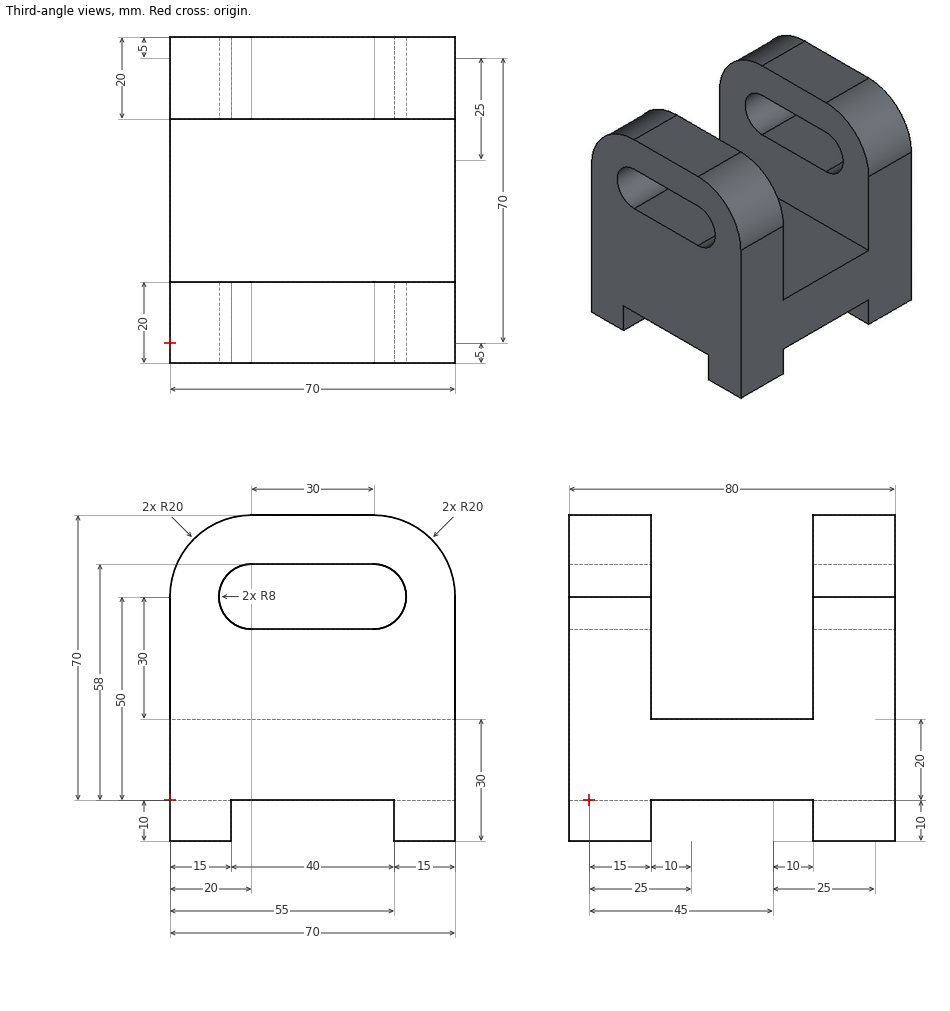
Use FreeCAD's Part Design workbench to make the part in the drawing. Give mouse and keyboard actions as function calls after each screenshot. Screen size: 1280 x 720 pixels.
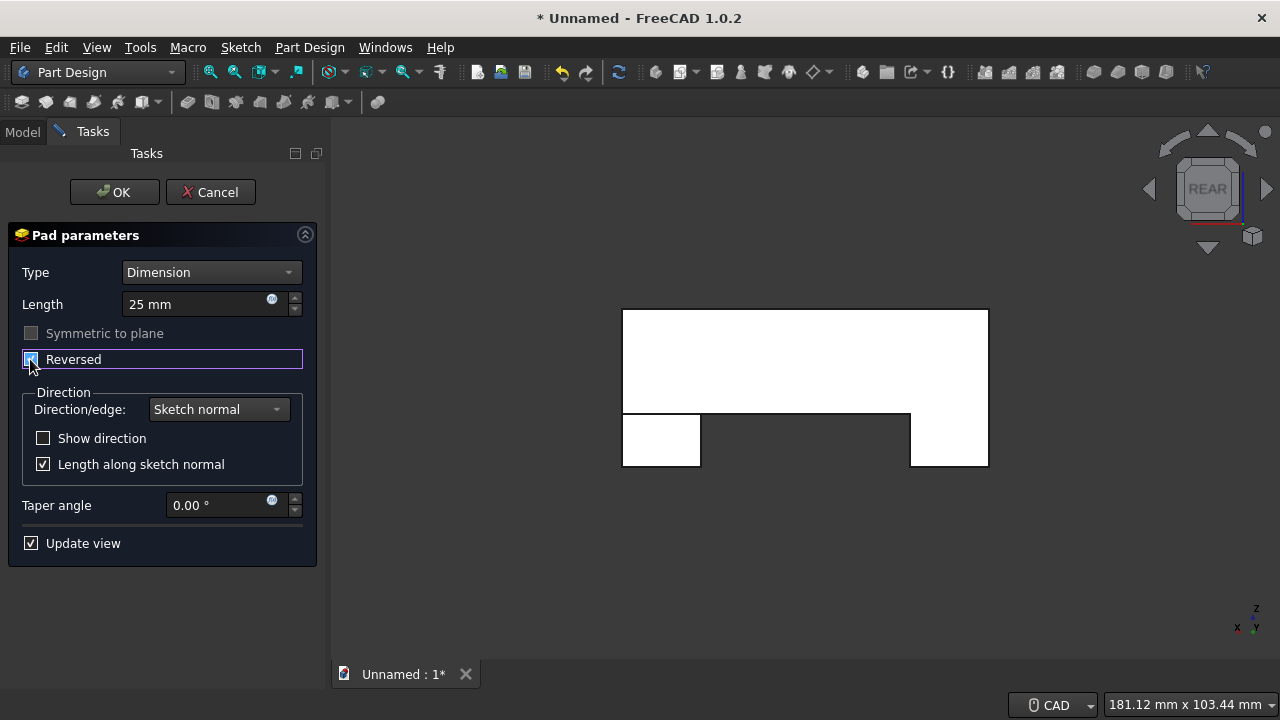
click(115, 192)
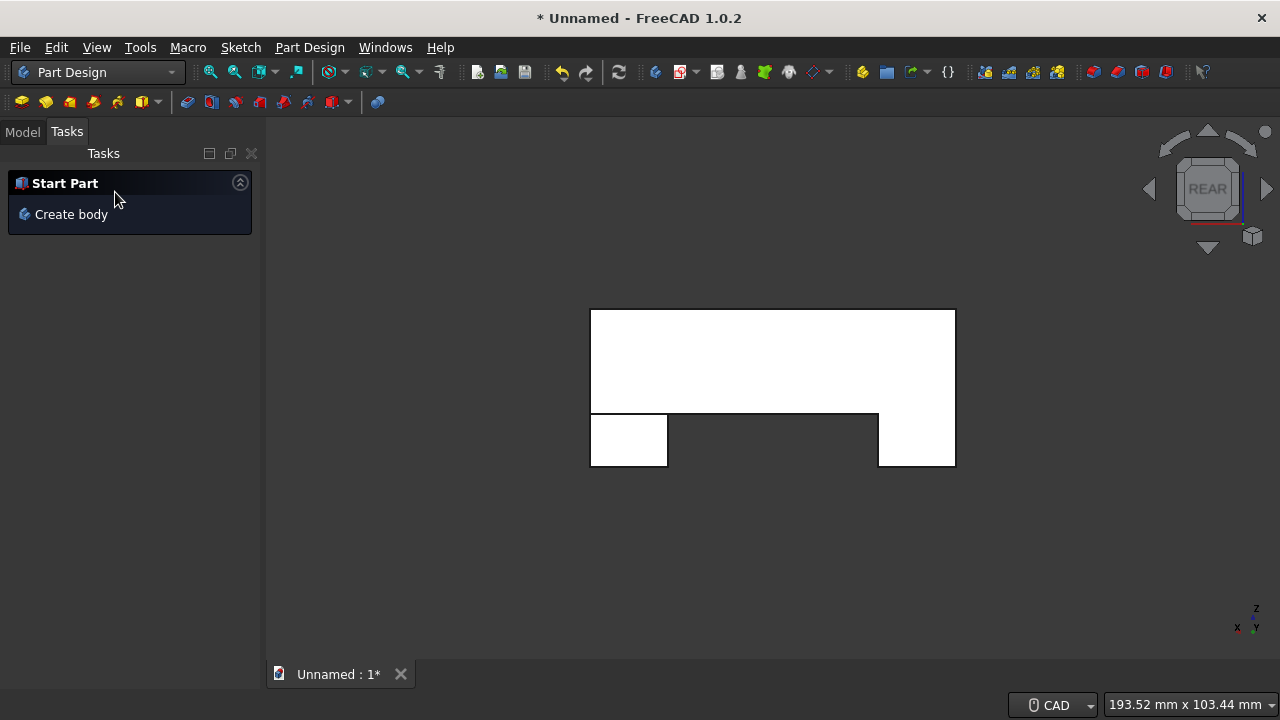
key(v)
key(f)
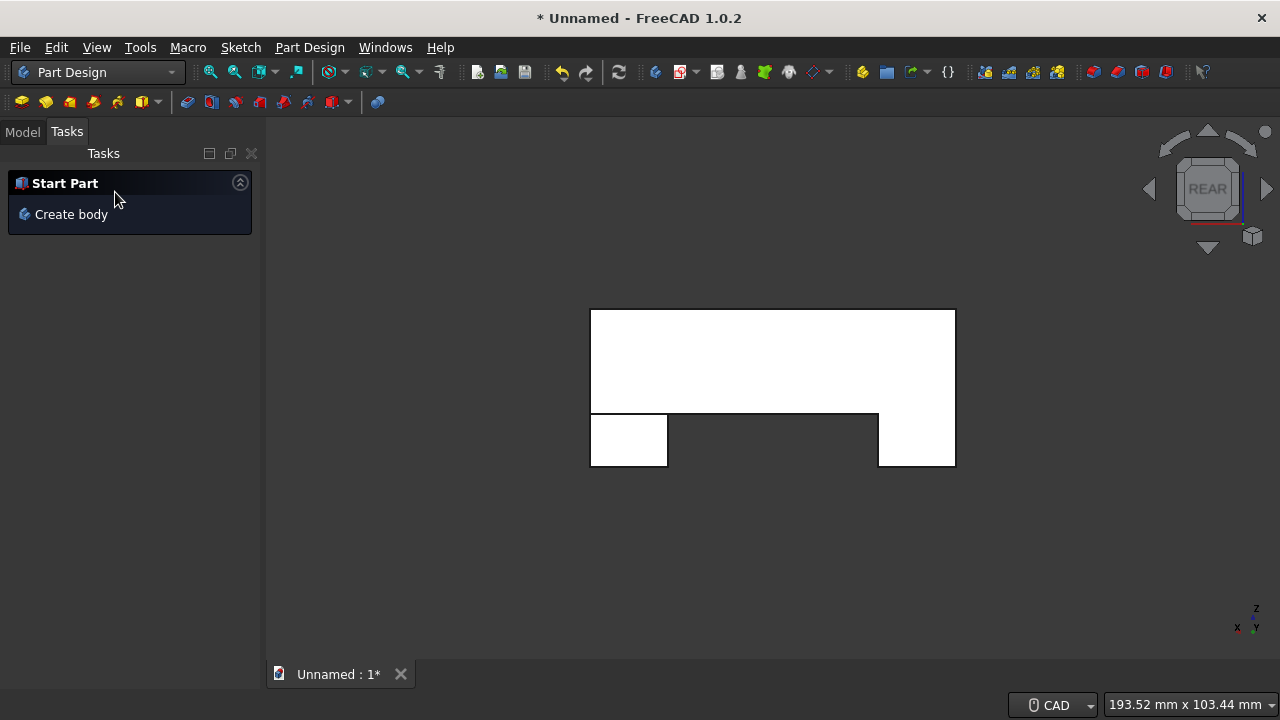
click(668, 365)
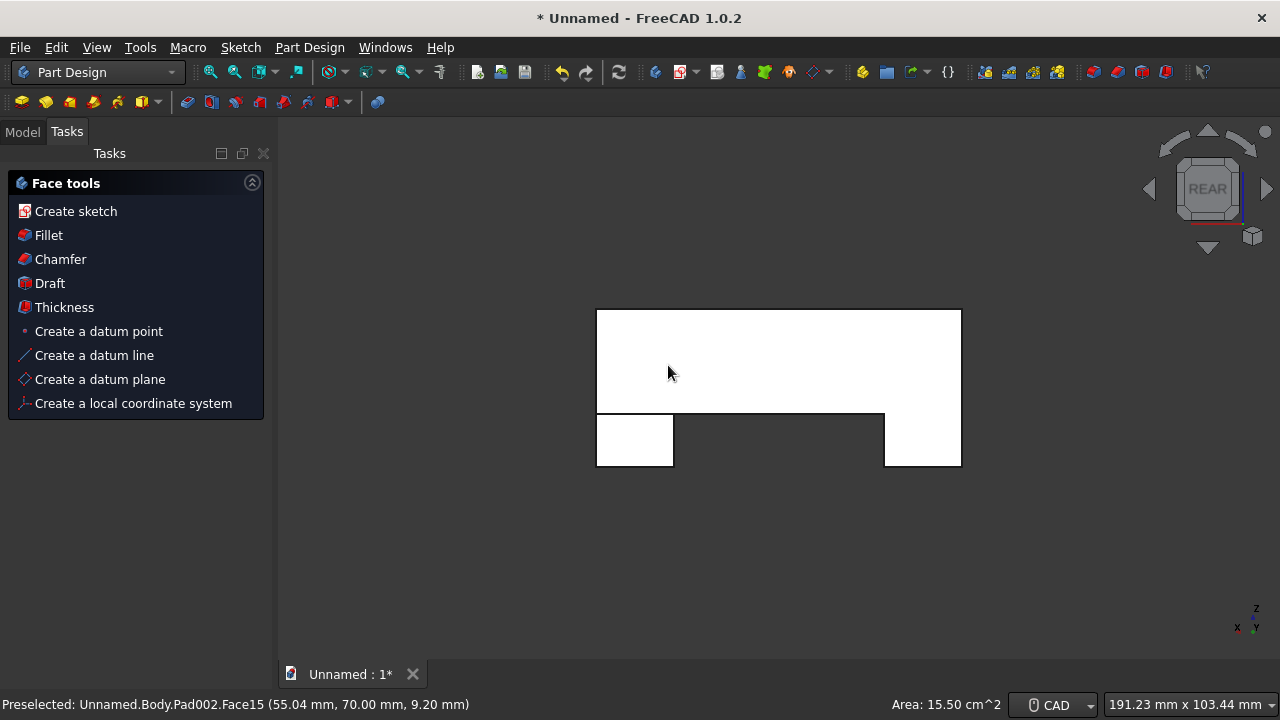
click(680, 72)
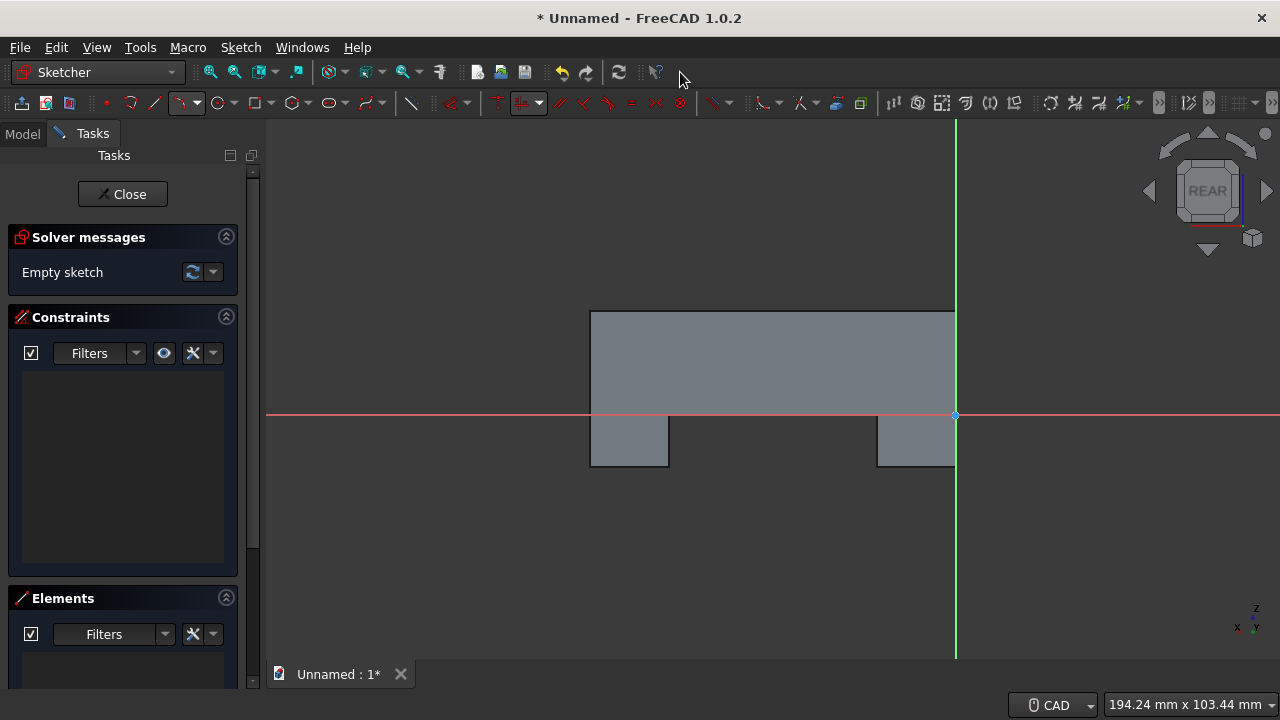
scroll(615, 452, up, 9)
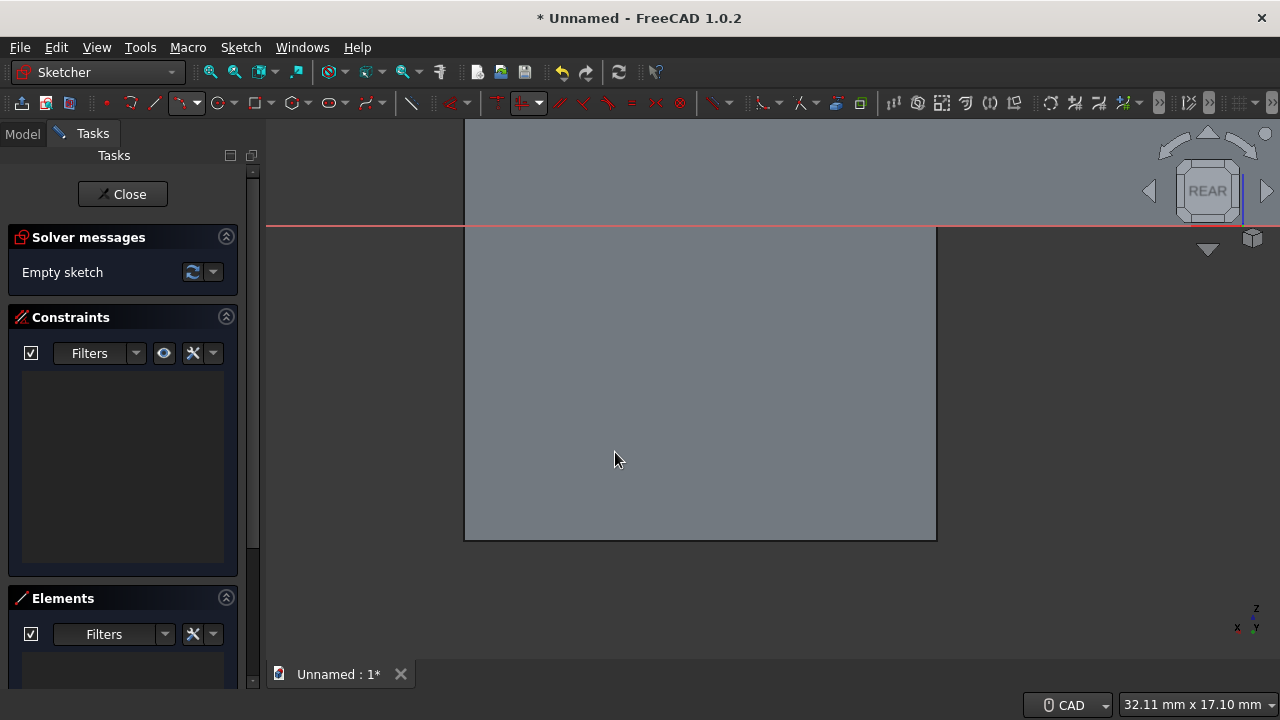
click(256, 104)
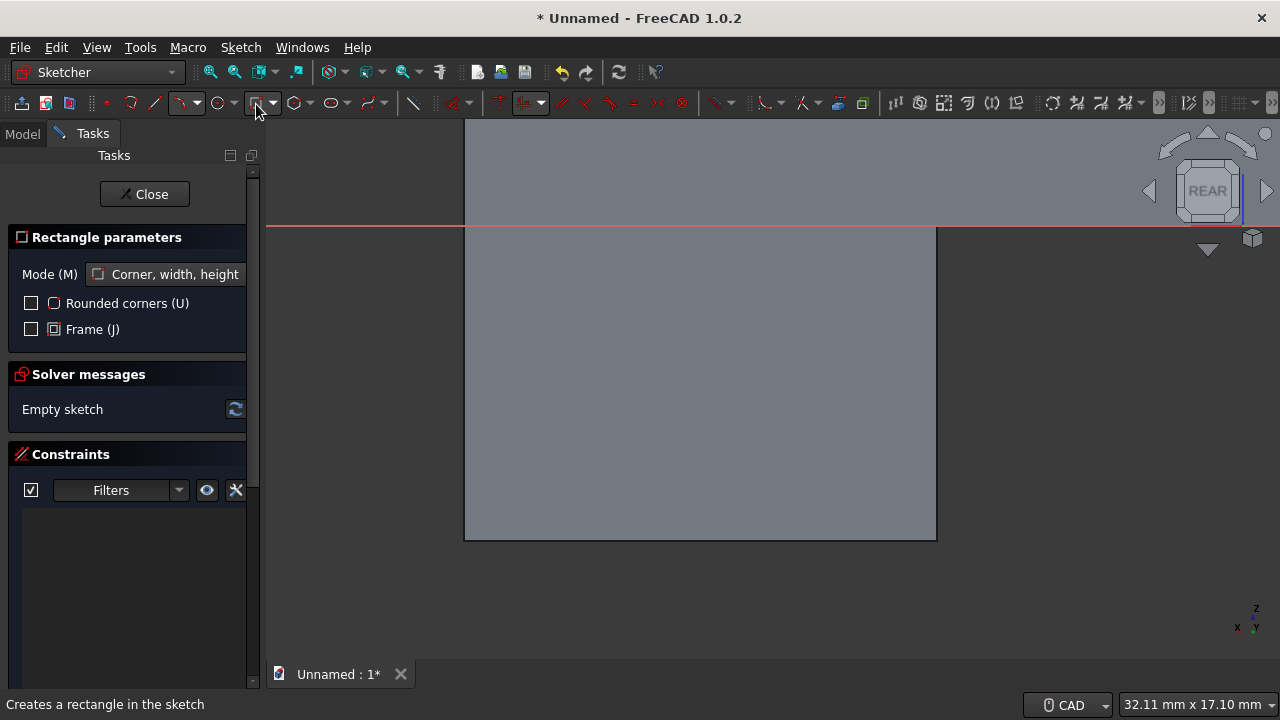
click(464, 226)
click(937, 541)
key(Escape)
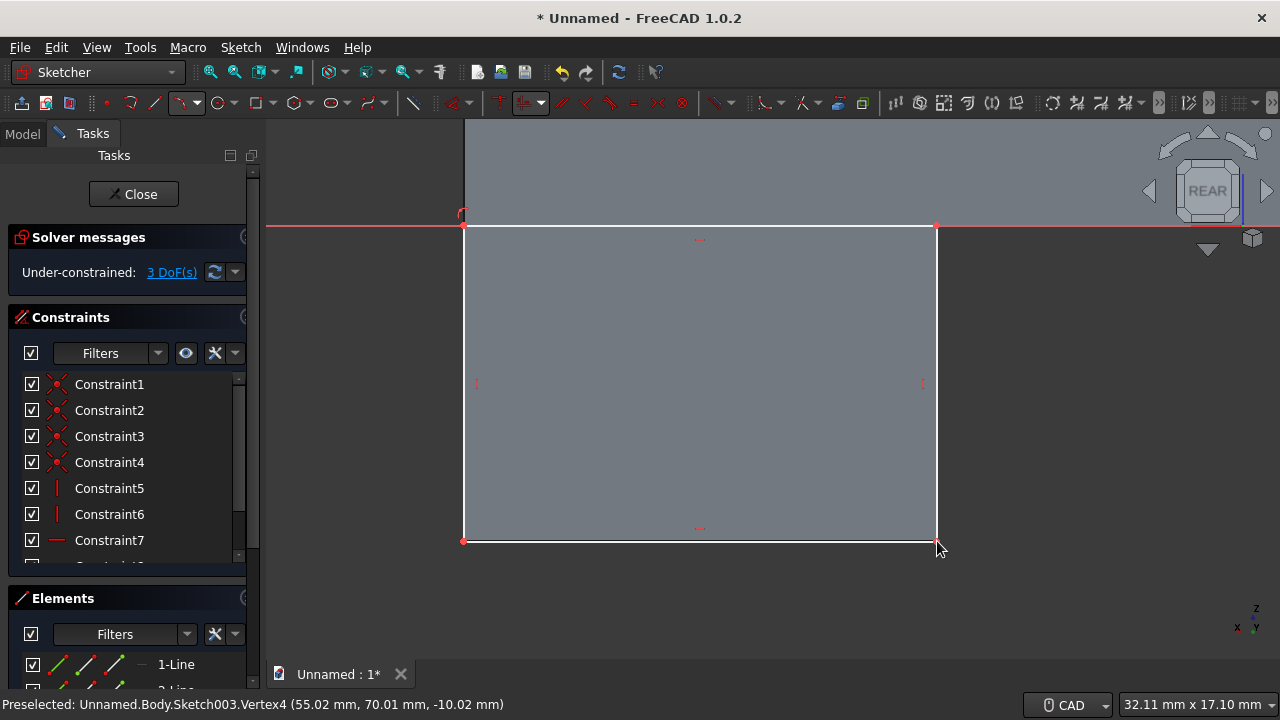
key(d)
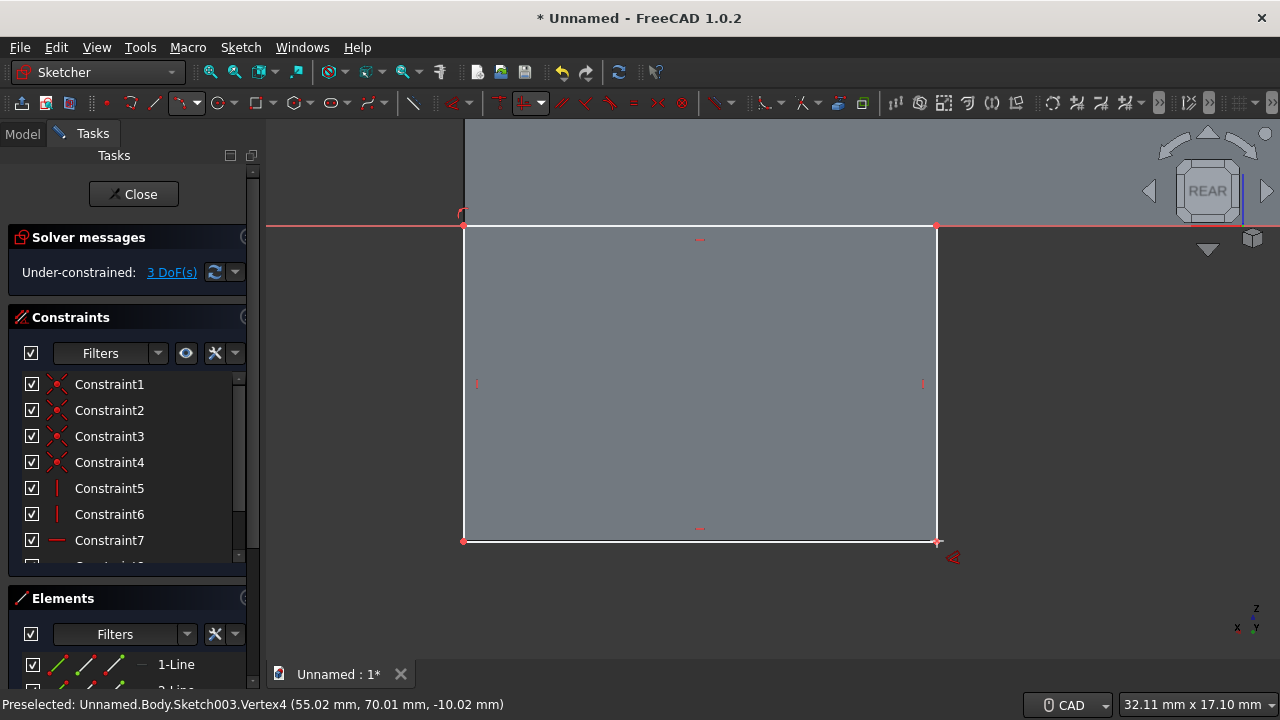
click(464, 321)
click(430, 384)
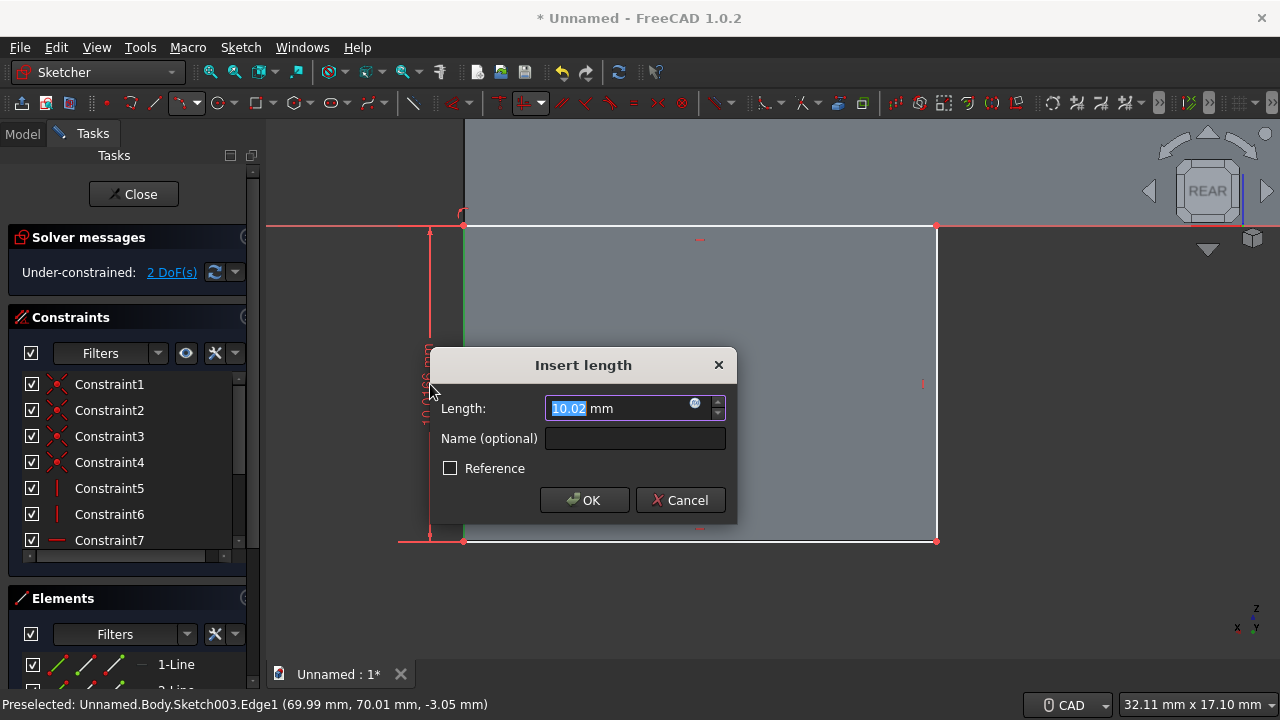
text(10)
key(Return)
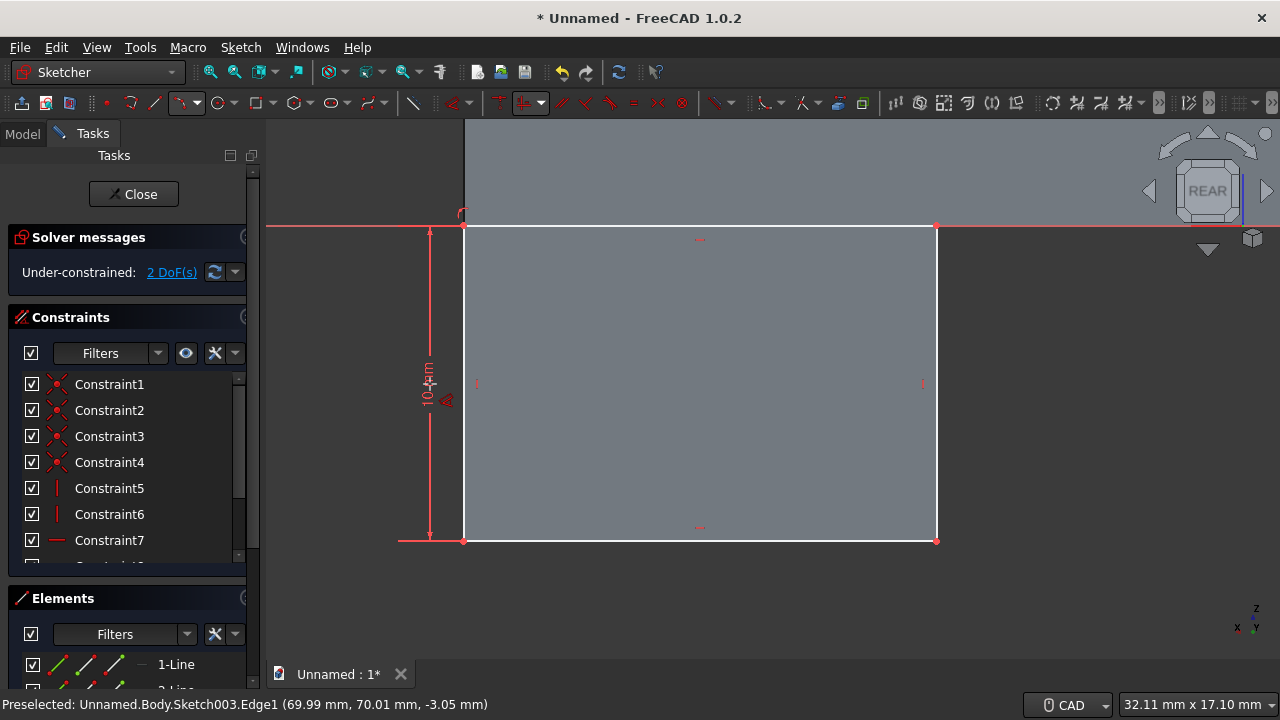
click(606, 541)
click(700, 575)